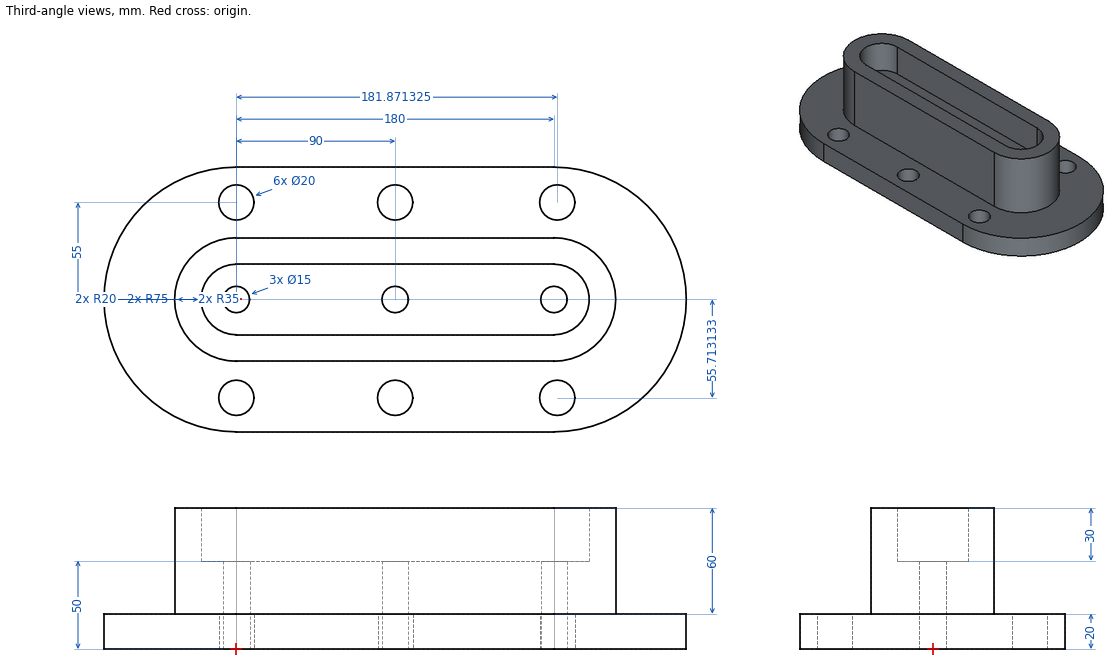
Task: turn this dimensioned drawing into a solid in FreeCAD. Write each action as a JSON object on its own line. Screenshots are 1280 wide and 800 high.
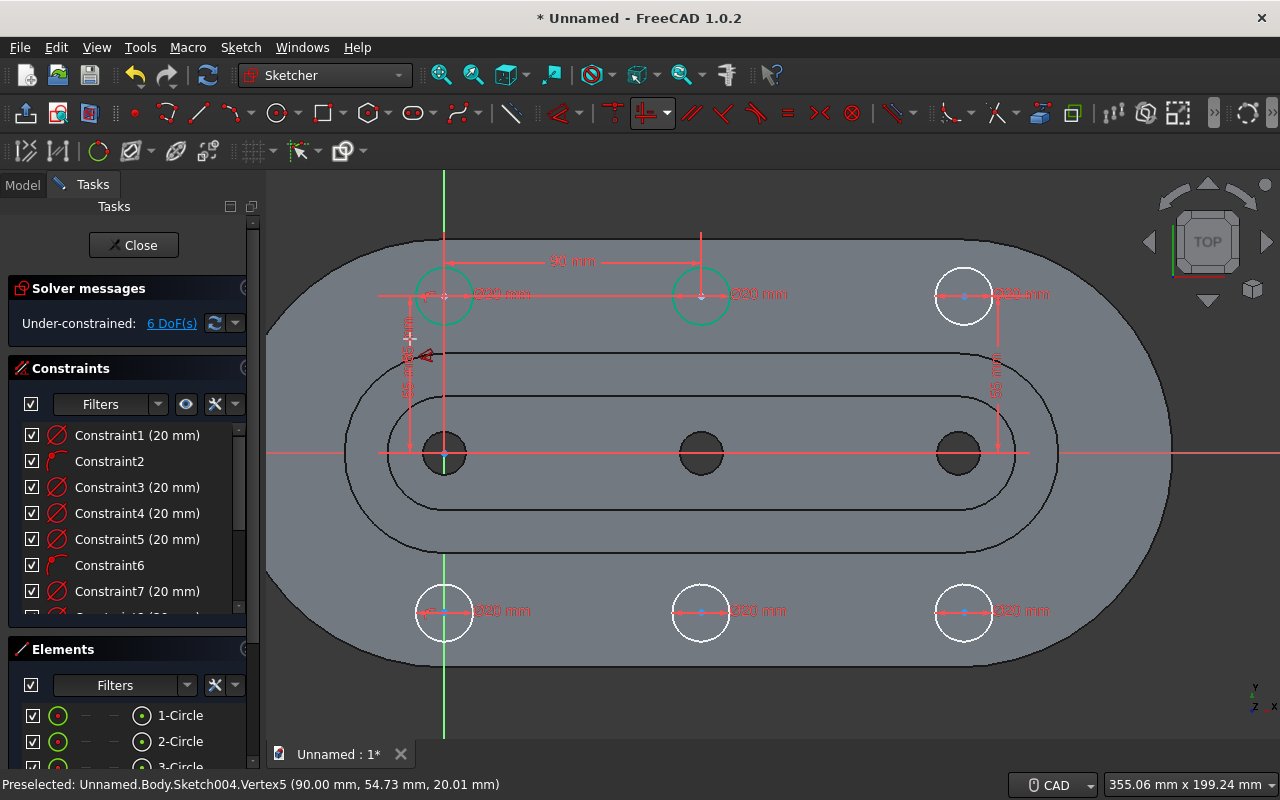
{"action": "left_click", "coordinate": [701, 613]}
{"action": "left_click", "coordinate": [573, 647]}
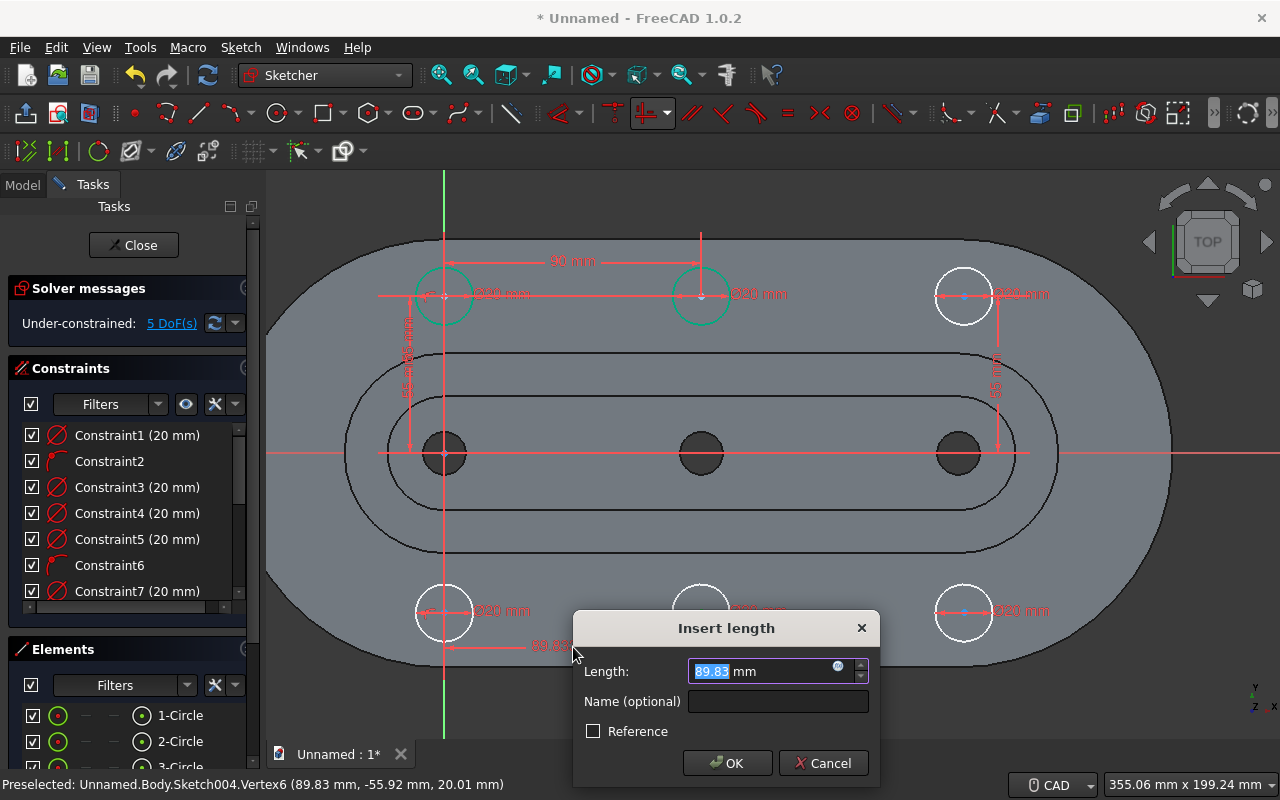
{"action": "type", "text": "90"}
{"action": "key", "text": "Return"}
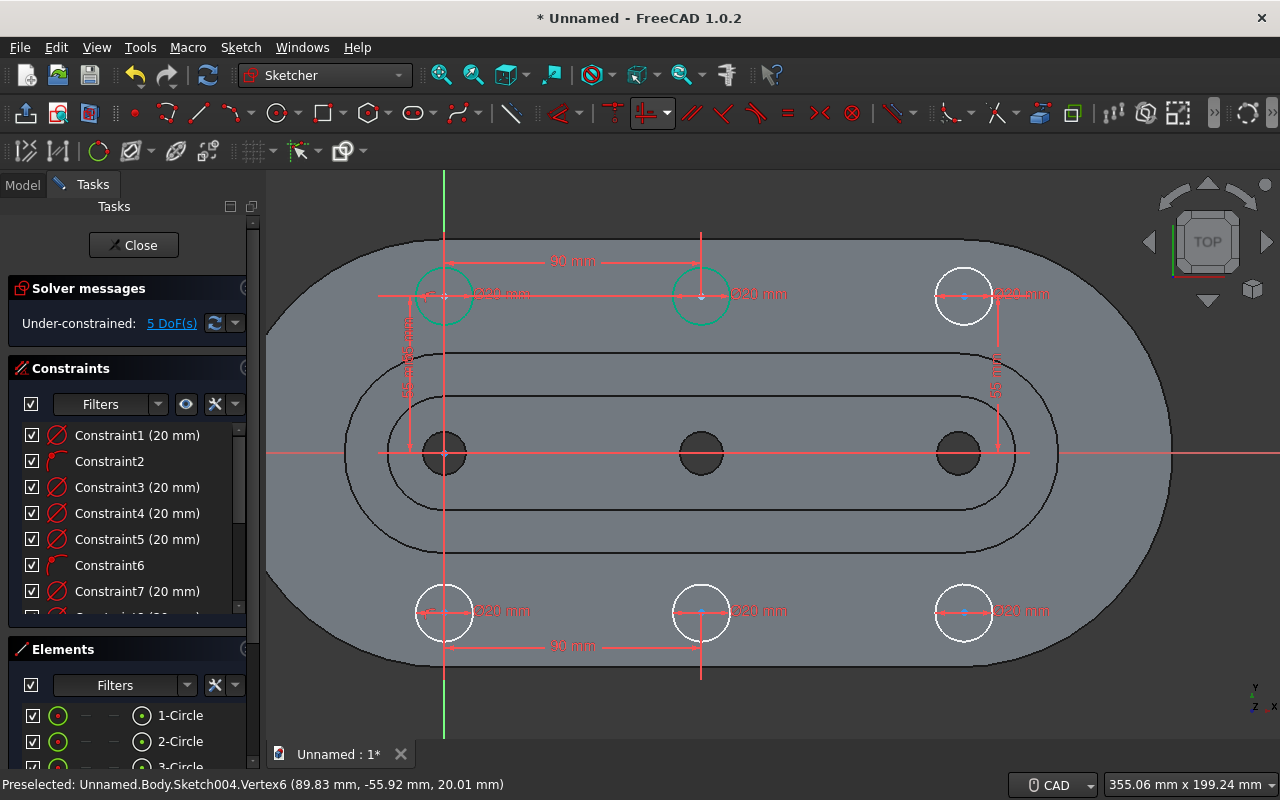
{"action": "left_click", "coordinate": [964, 613]}
{"action": "left_click", "coordinate": [998, 533]}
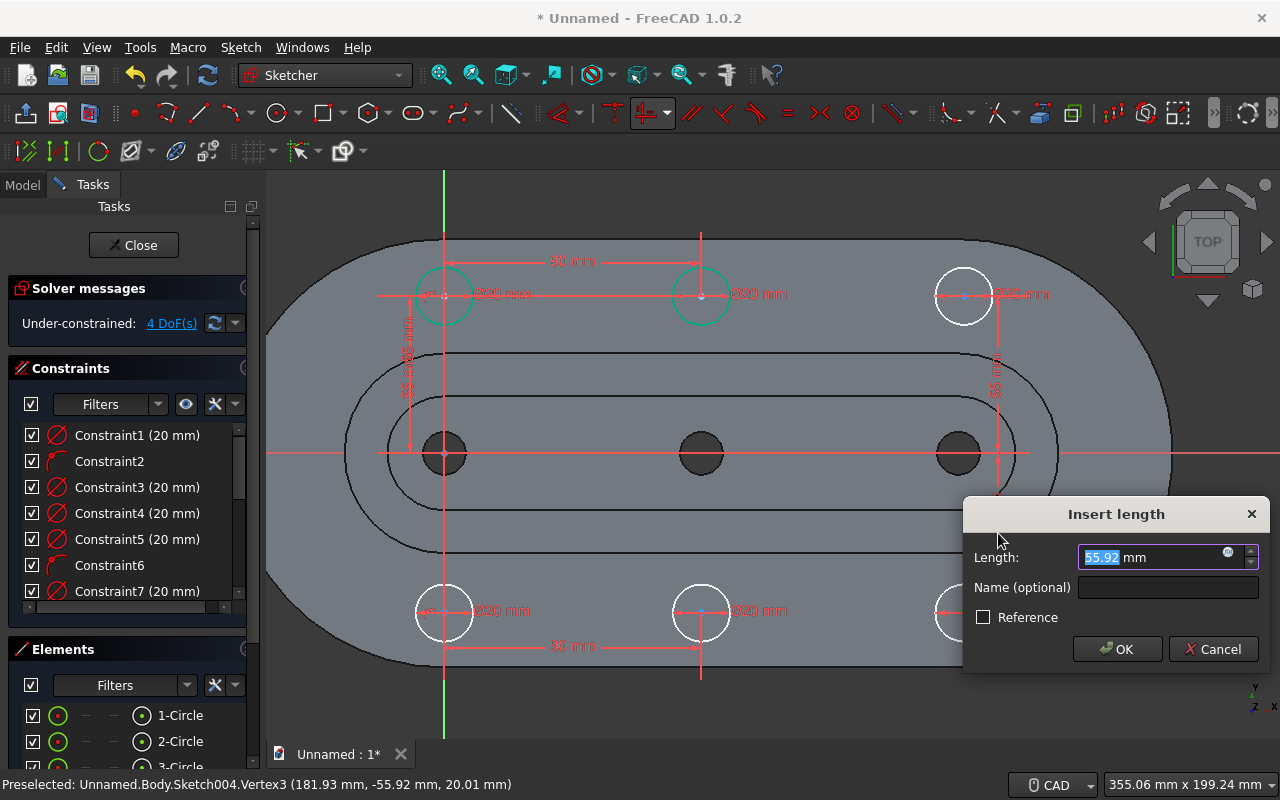
{"action": "type", "text": "55.713133"}
{"action": "key", "text": "Return"}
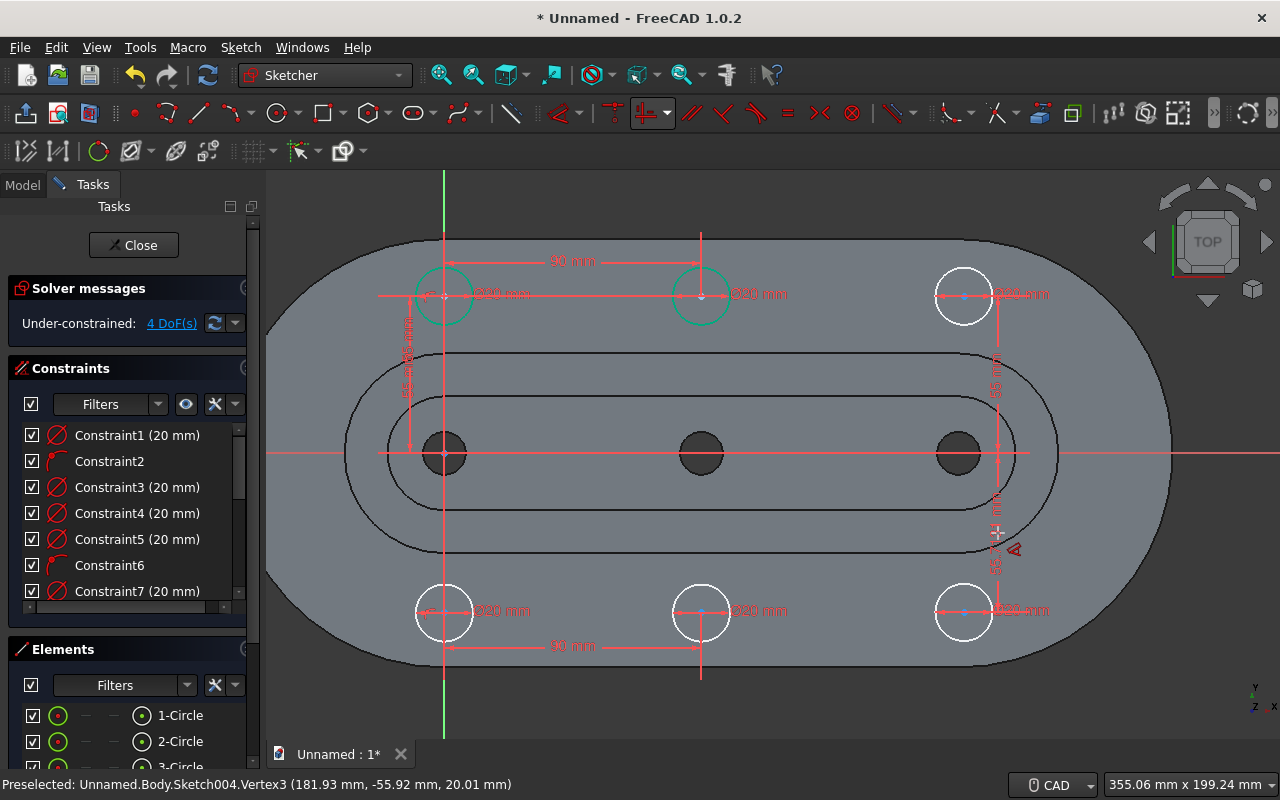
{"action": "left_click", "coordinate": [444, 613]}
{"action": "left_click", "coordinate": [410, 533]}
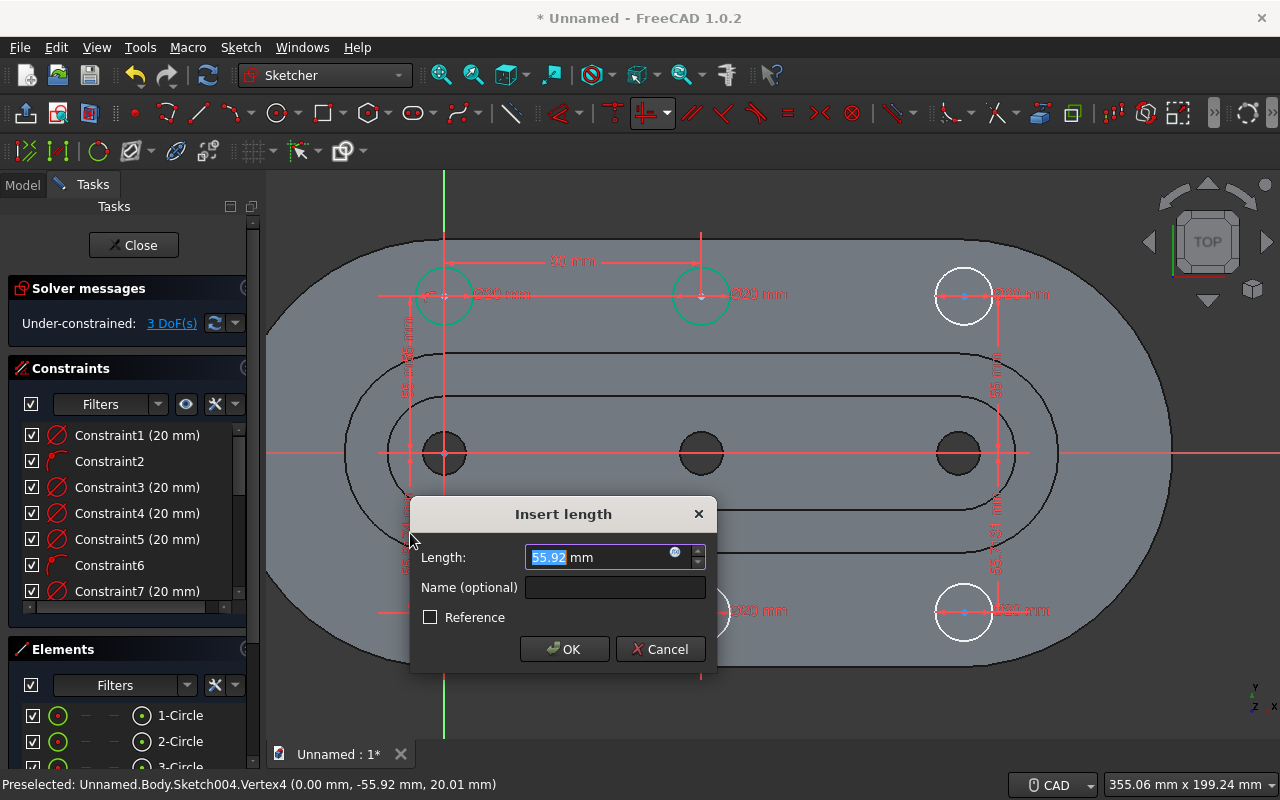
{"action": "type", "text": "55.713133"}
{"action": "key", "text": "Return"}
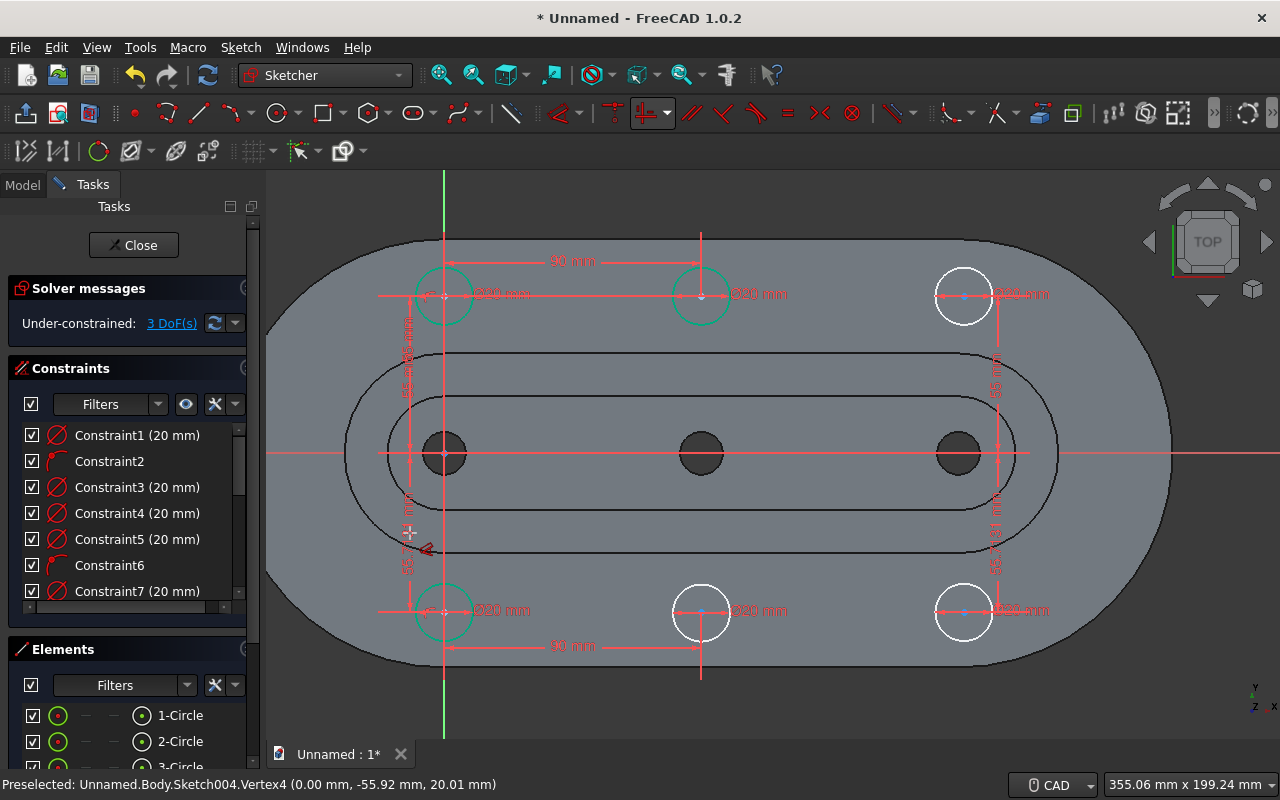
{"action": "left_click", "coordinate": [701, 613]}
{"action": "left_click", "coordinate": [410, 496]}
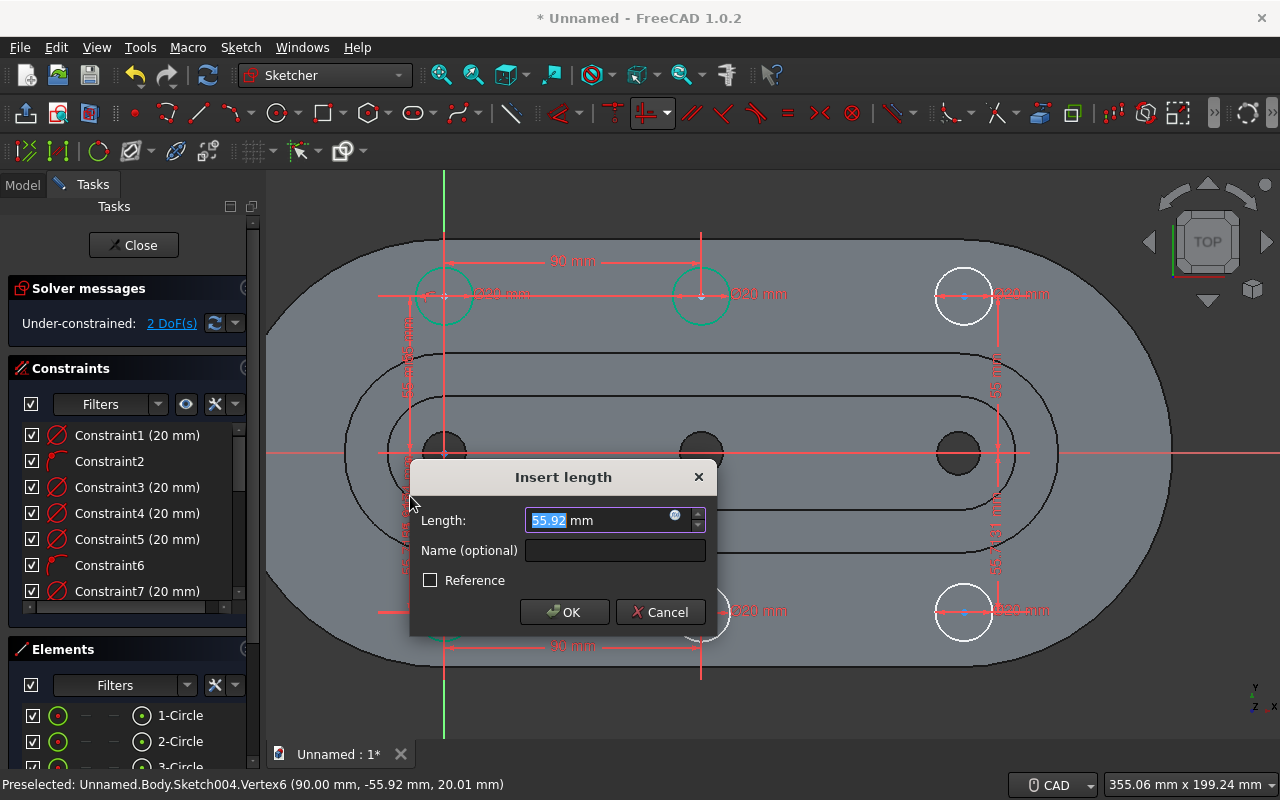
{"action": "type", "text": "55.713133"}
{"action": "key", "text": "Return"}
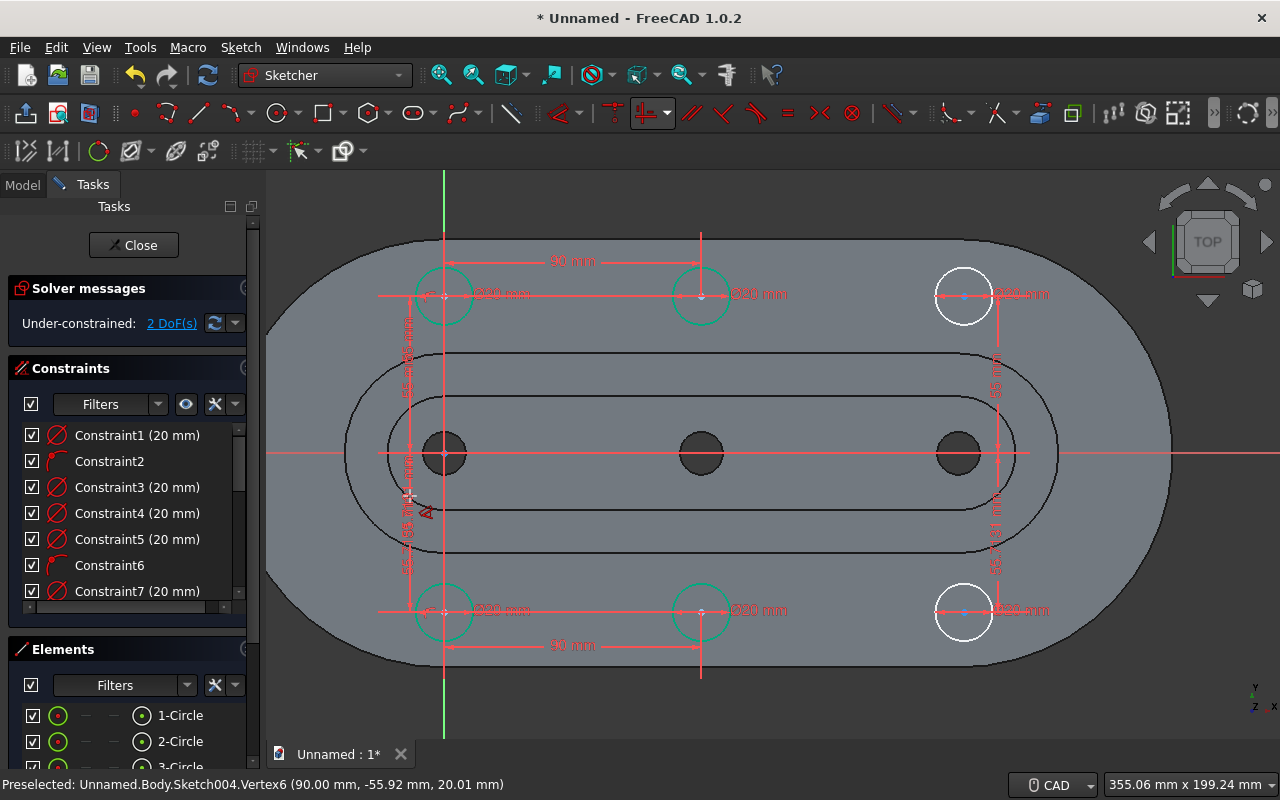
{"action": "left_click", "coordinate": [964, 296]}
{"action": "left_click", "coordinate": [824, 262]}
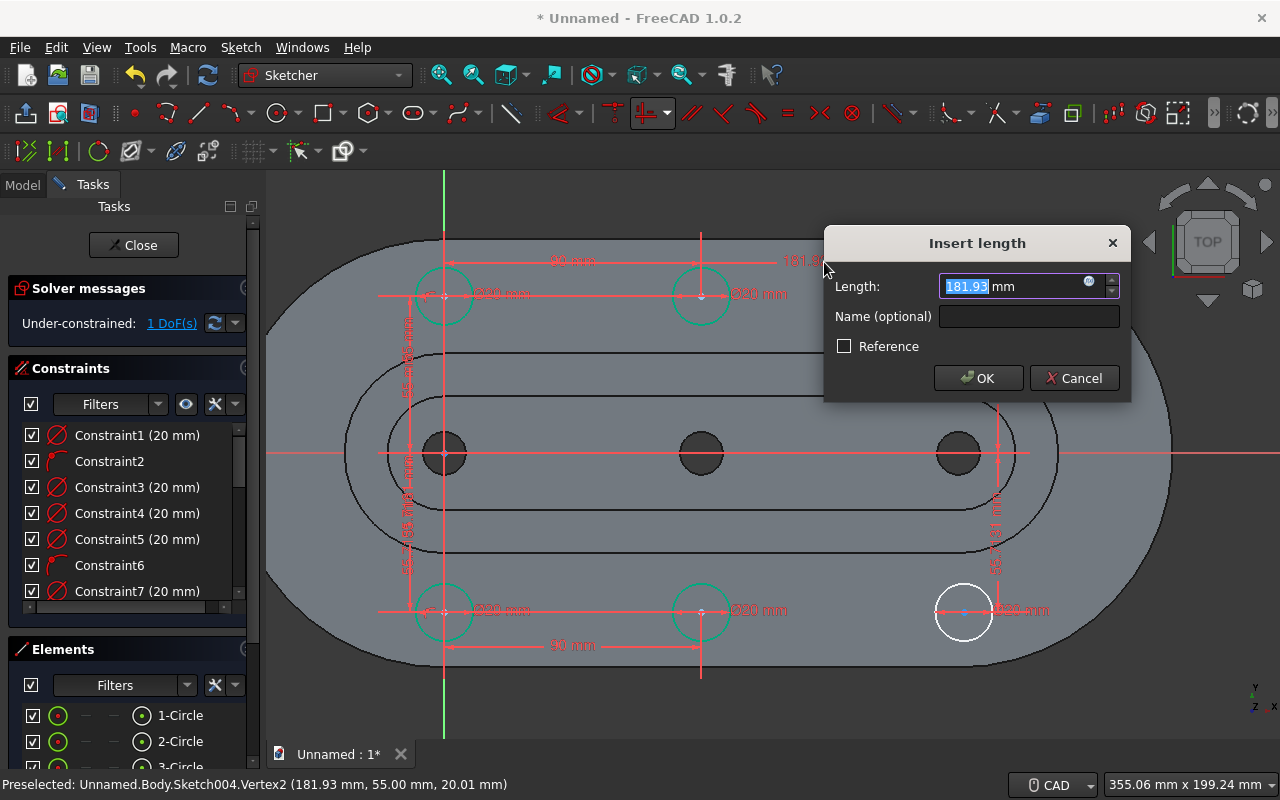
{"action": "type", "text": "181.871325"}
{"action": "key", "text": "Return"}